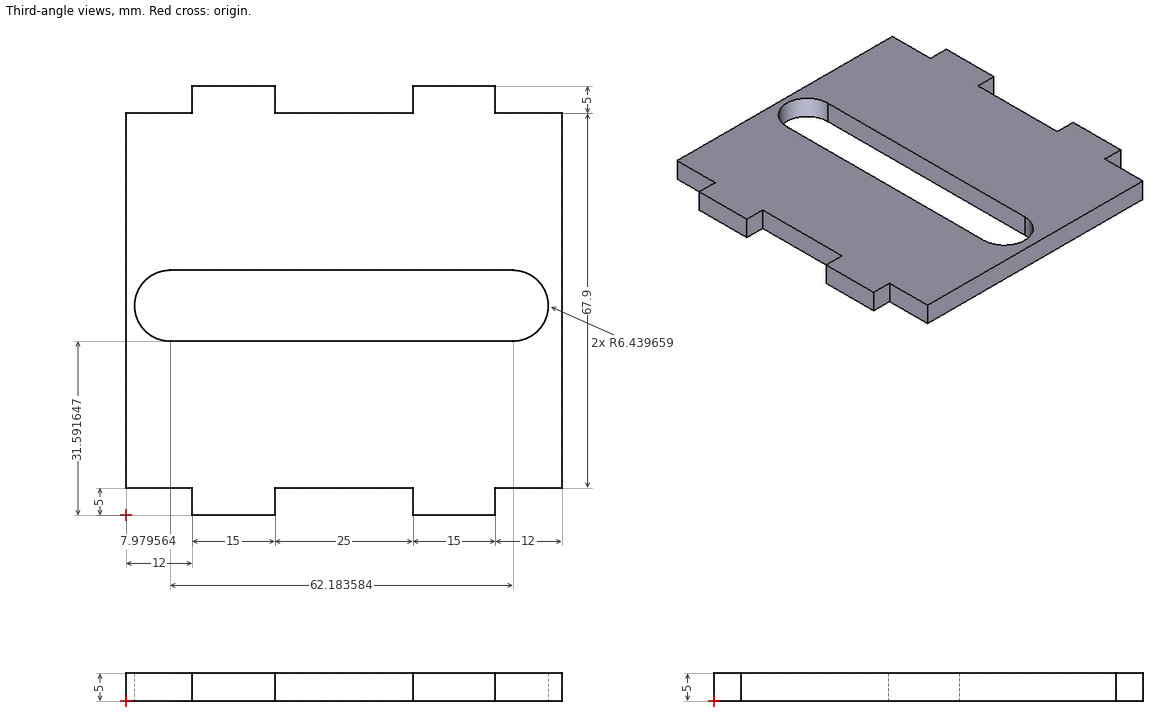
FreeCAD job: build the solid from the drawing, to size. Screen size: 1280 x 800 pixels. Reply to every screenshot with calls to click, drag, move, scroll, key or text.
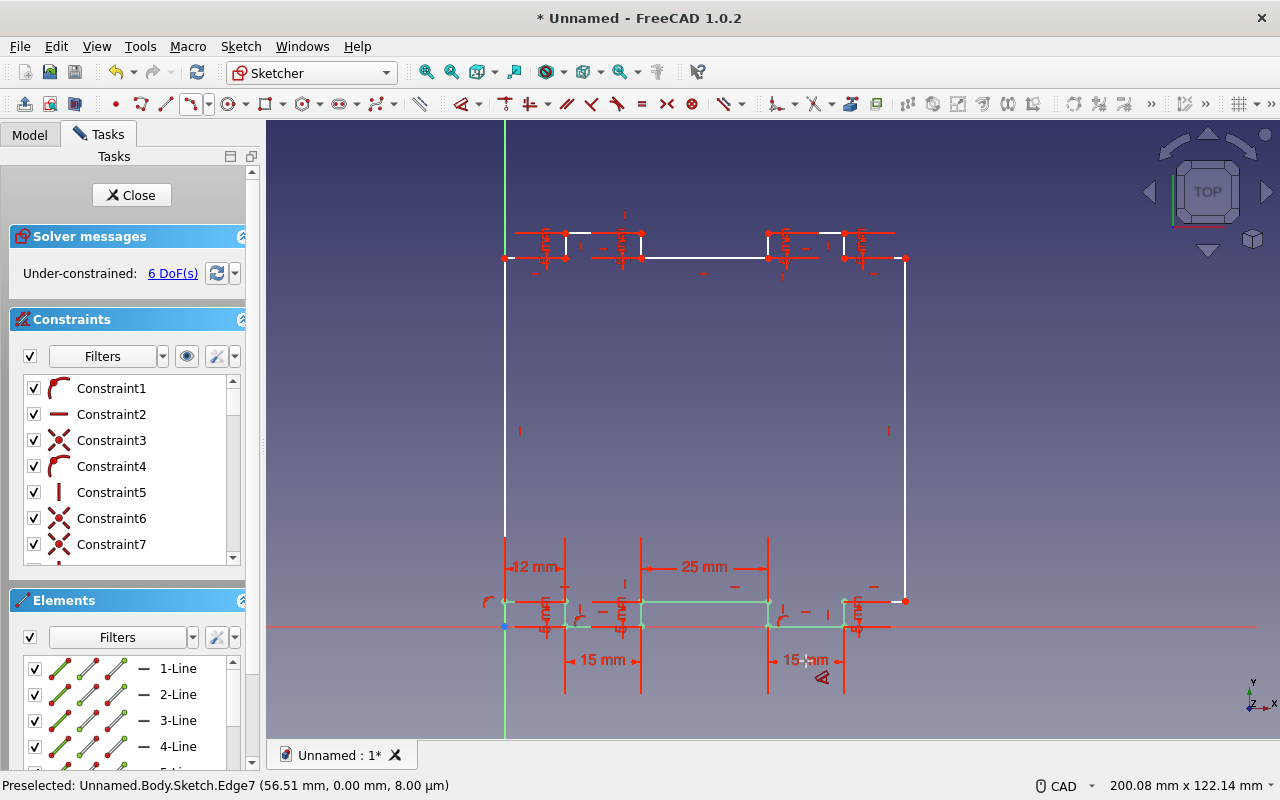
click(862, 602)
click(875, 568)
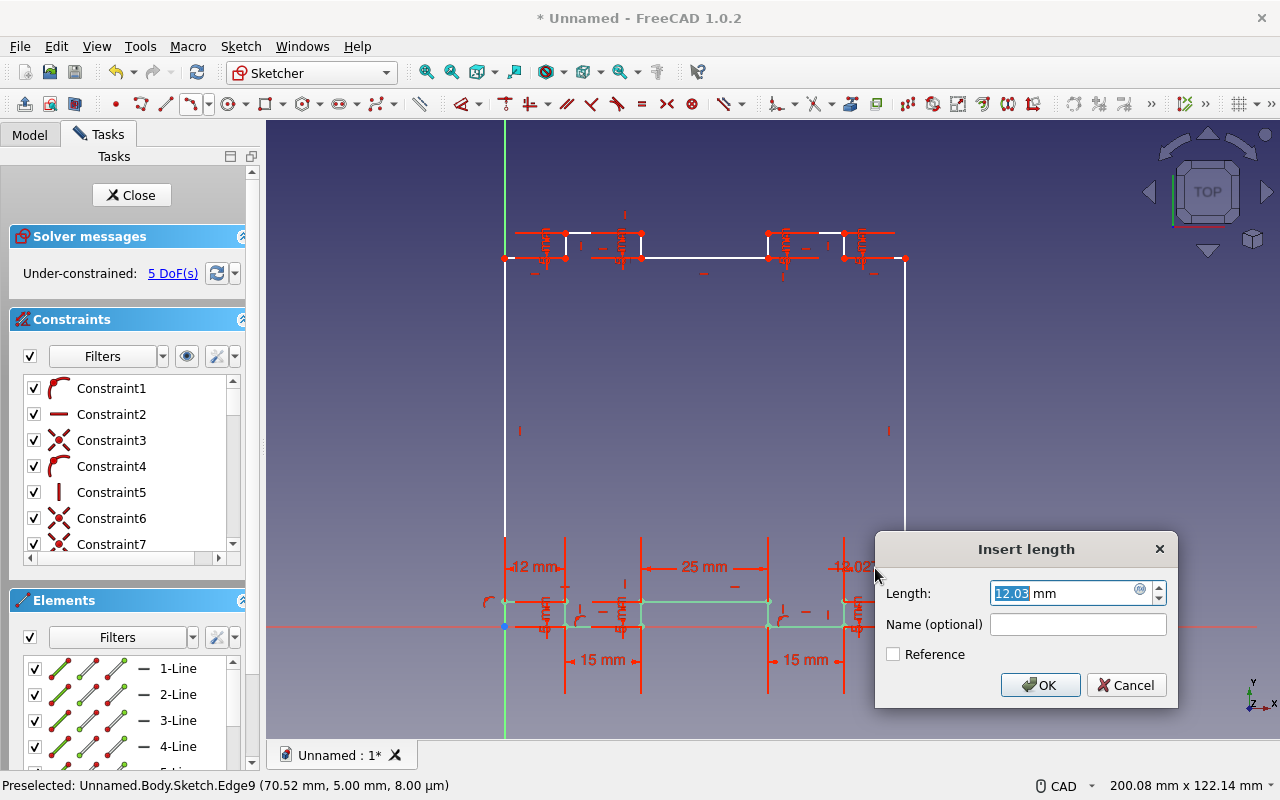
text(12)
key(Return)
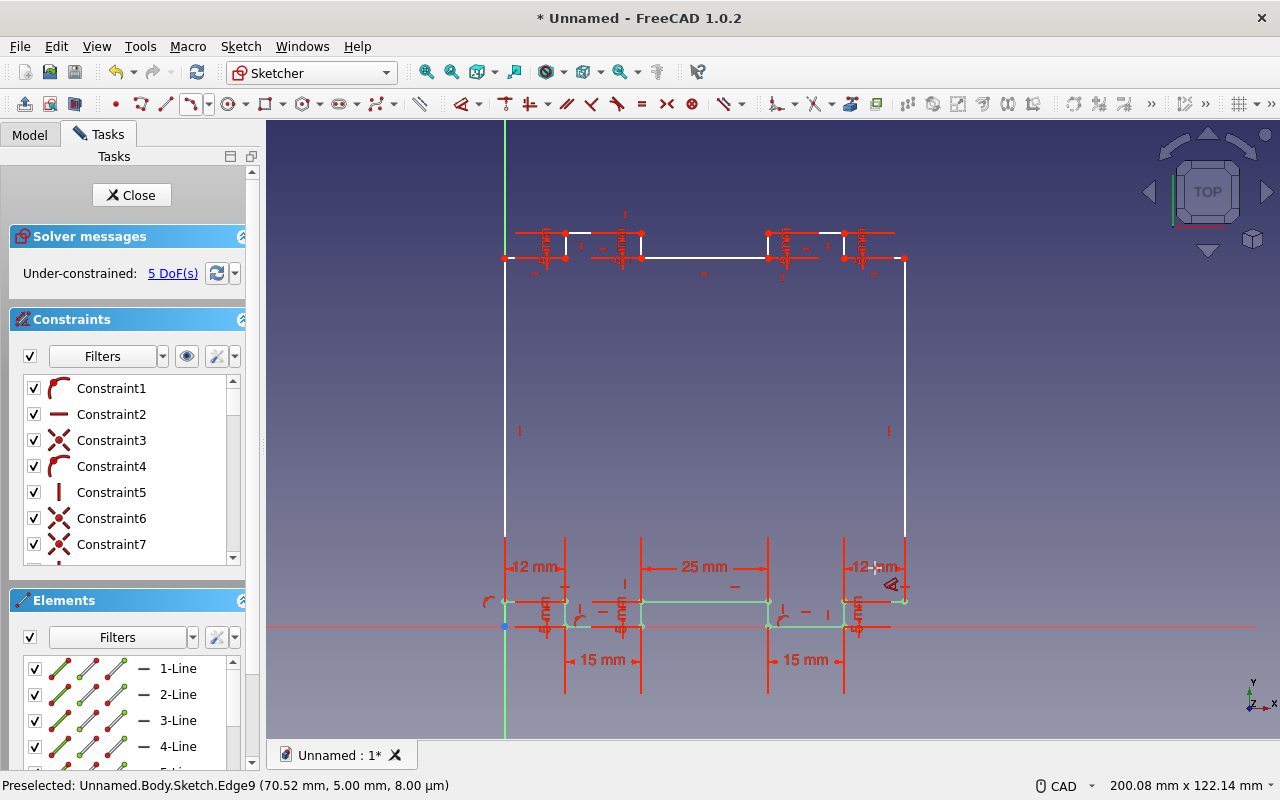
click(887, 258)
click(874, 224)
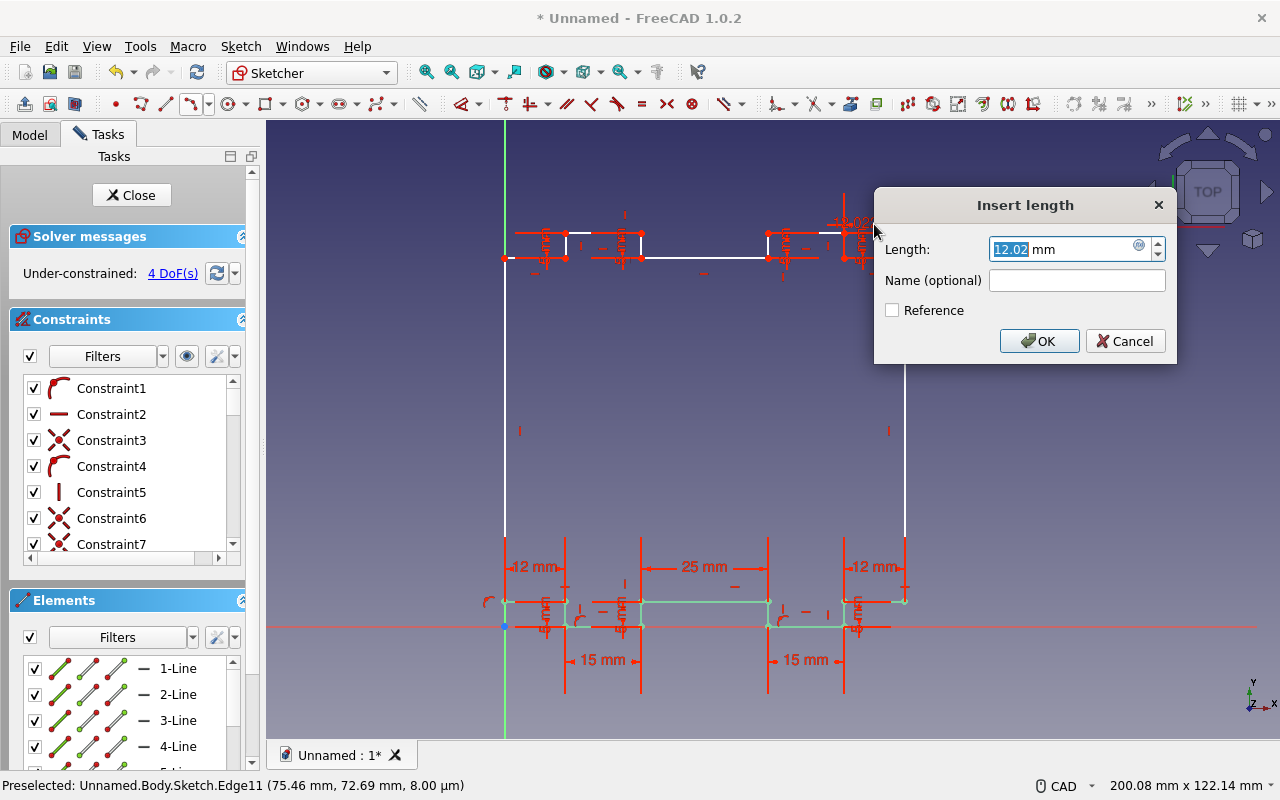
text(12)
key(Return)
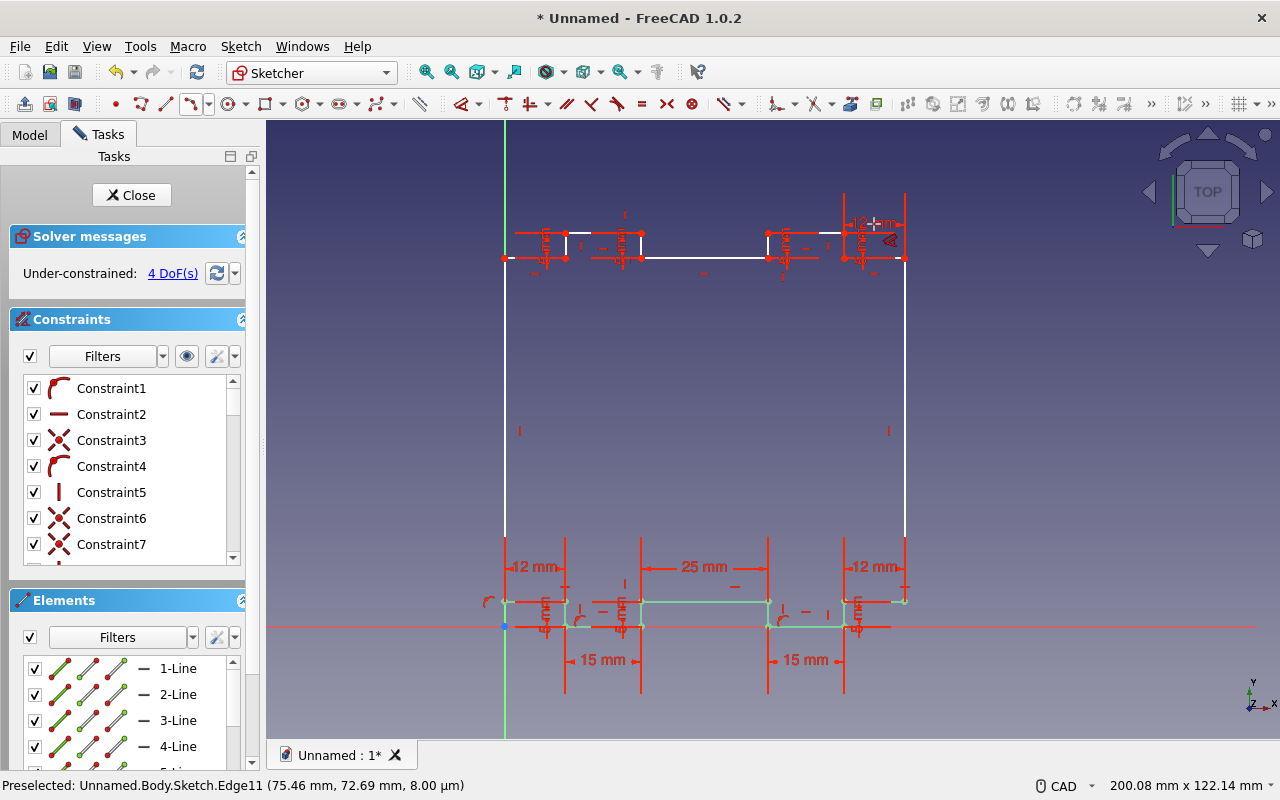
click(821, 233)
click(806, 199)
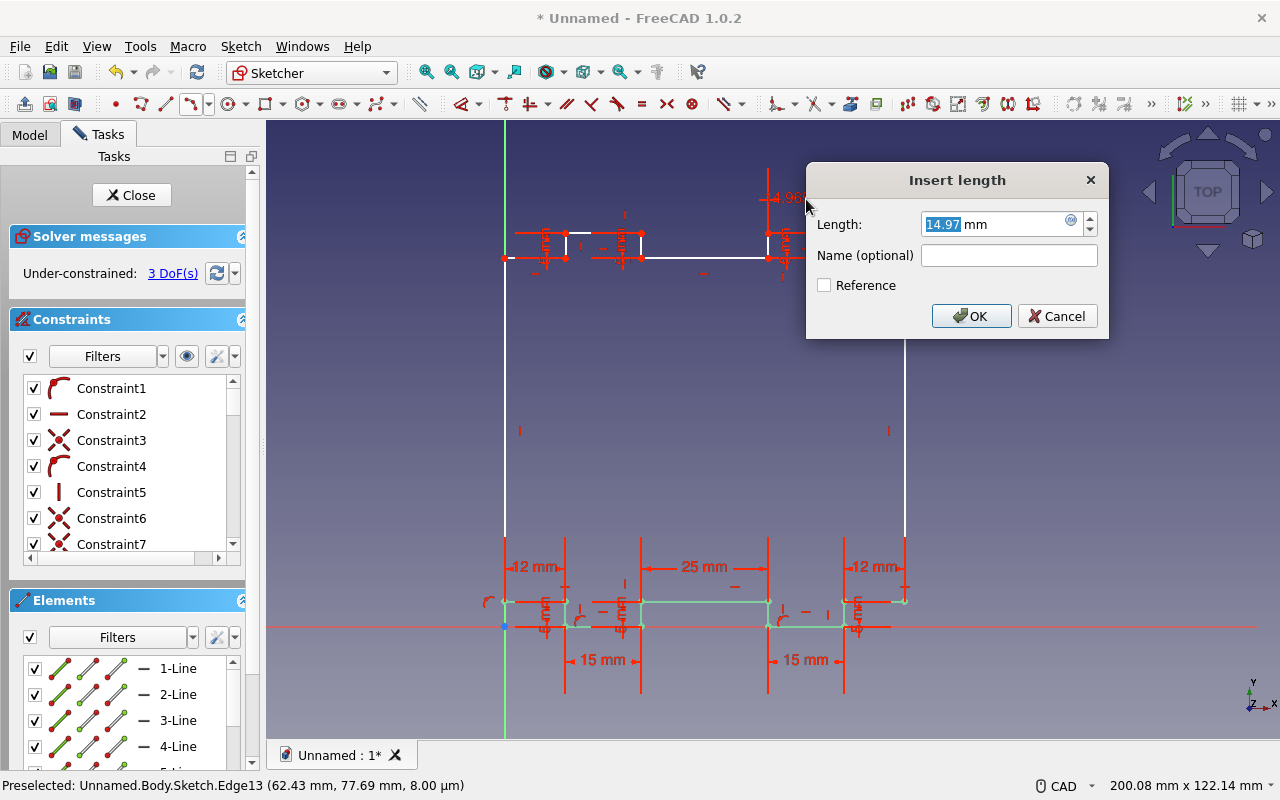
text(15)
key(Return)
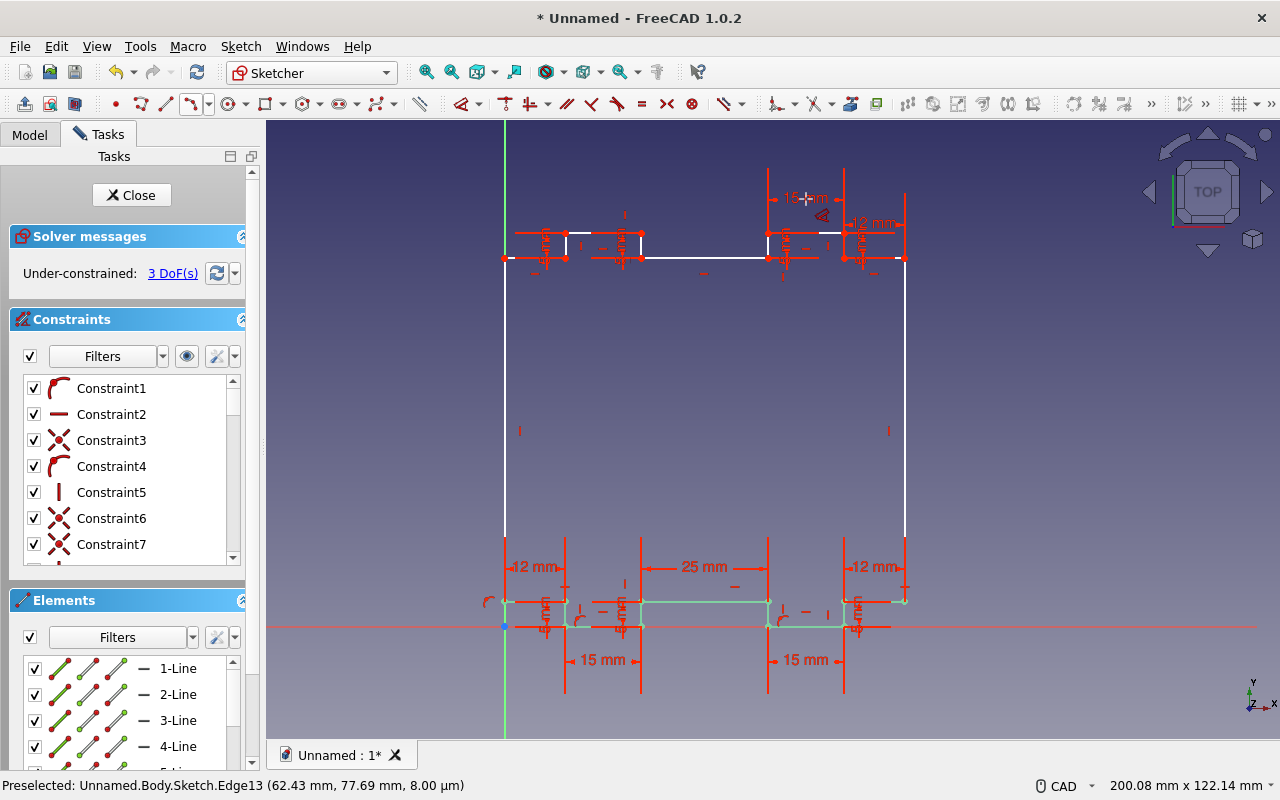
click(730, 258)
click(705, 224)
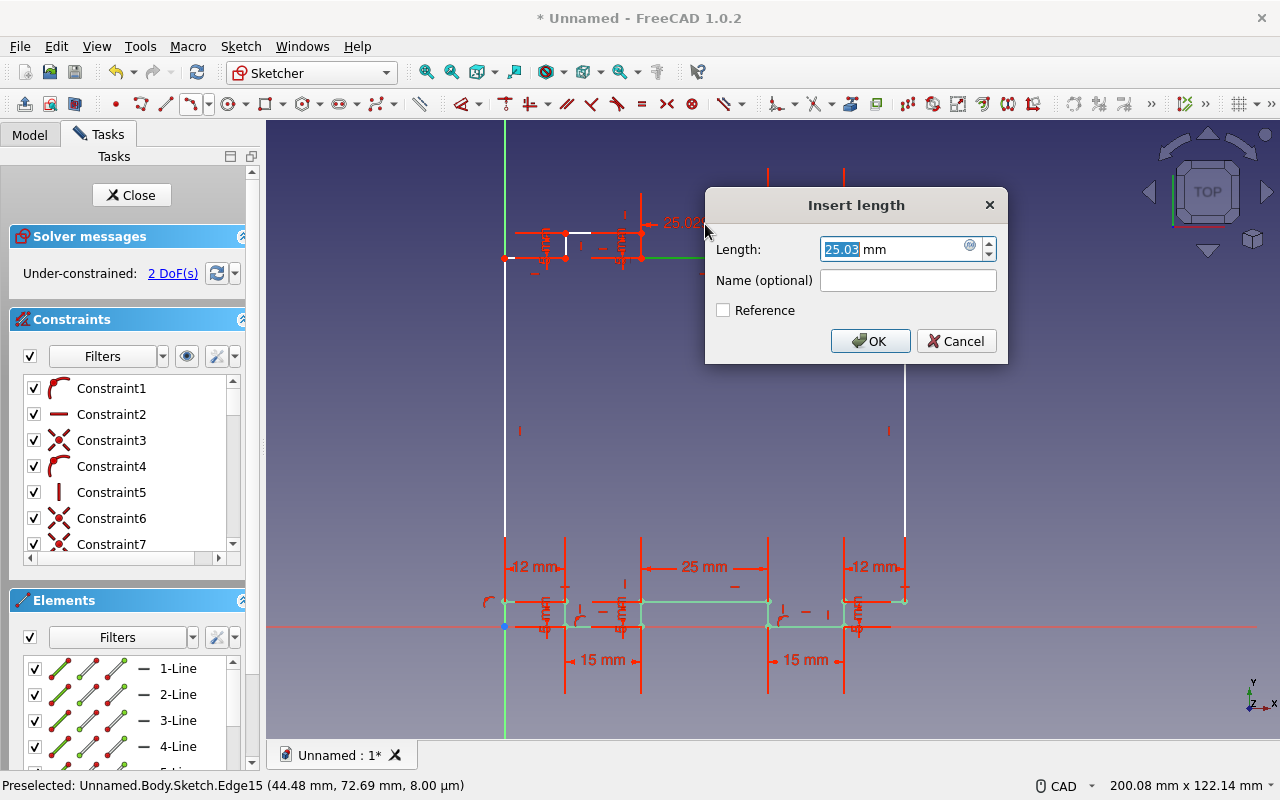
text(25)
key(Return)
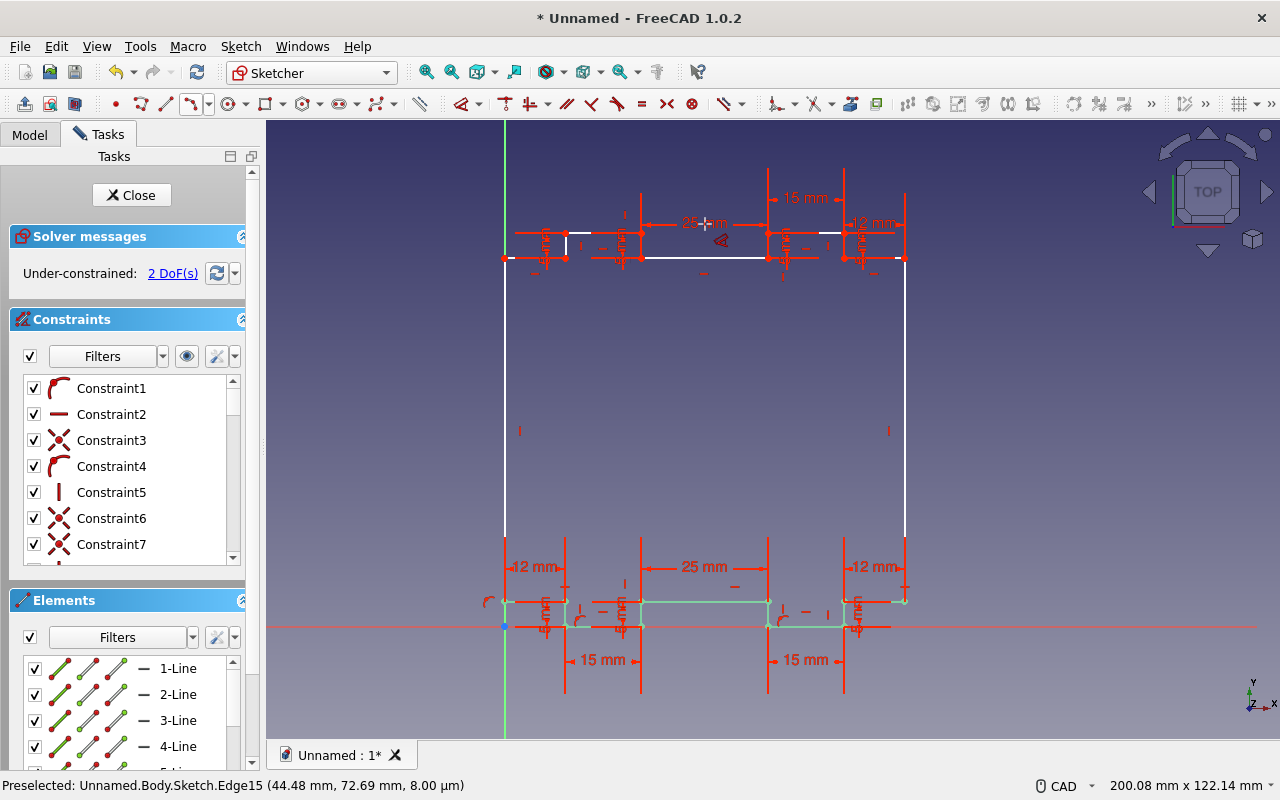
click(619, 233)
click(603, 199)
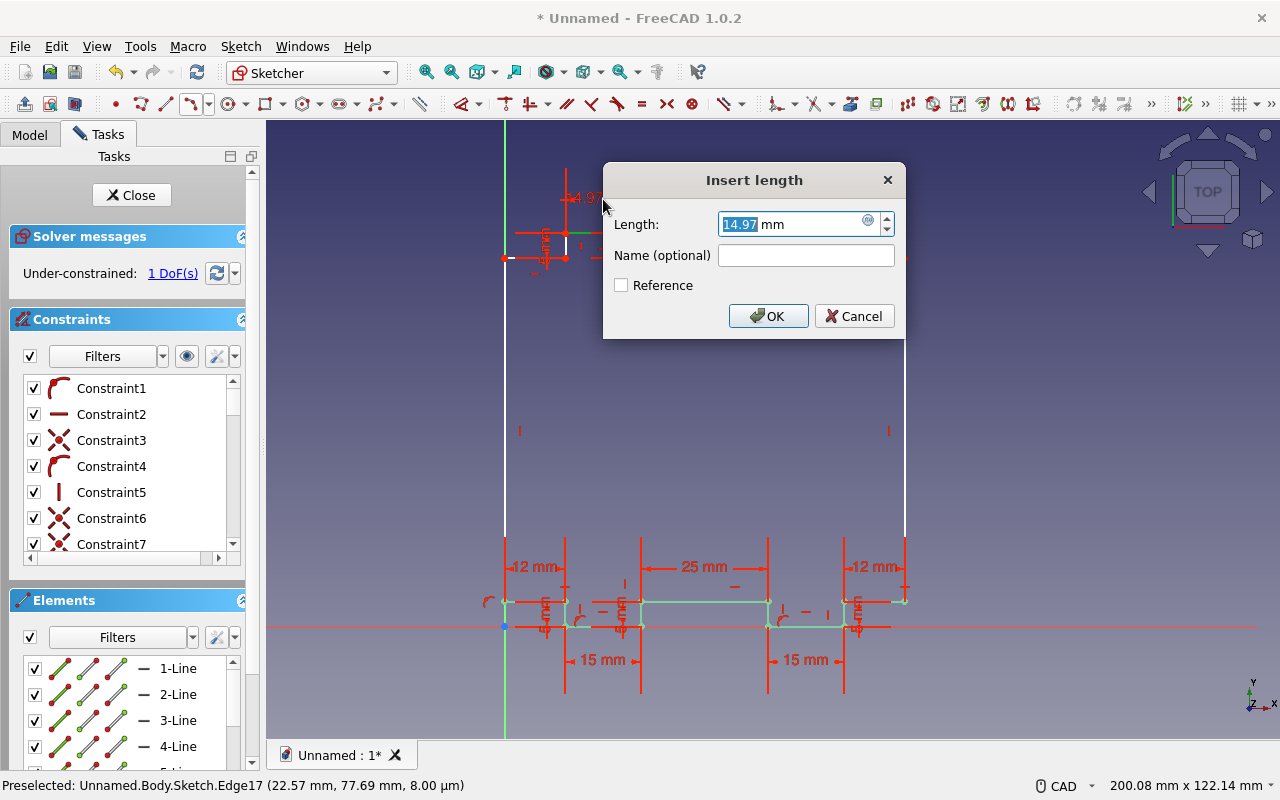
text(15)
key(Return)